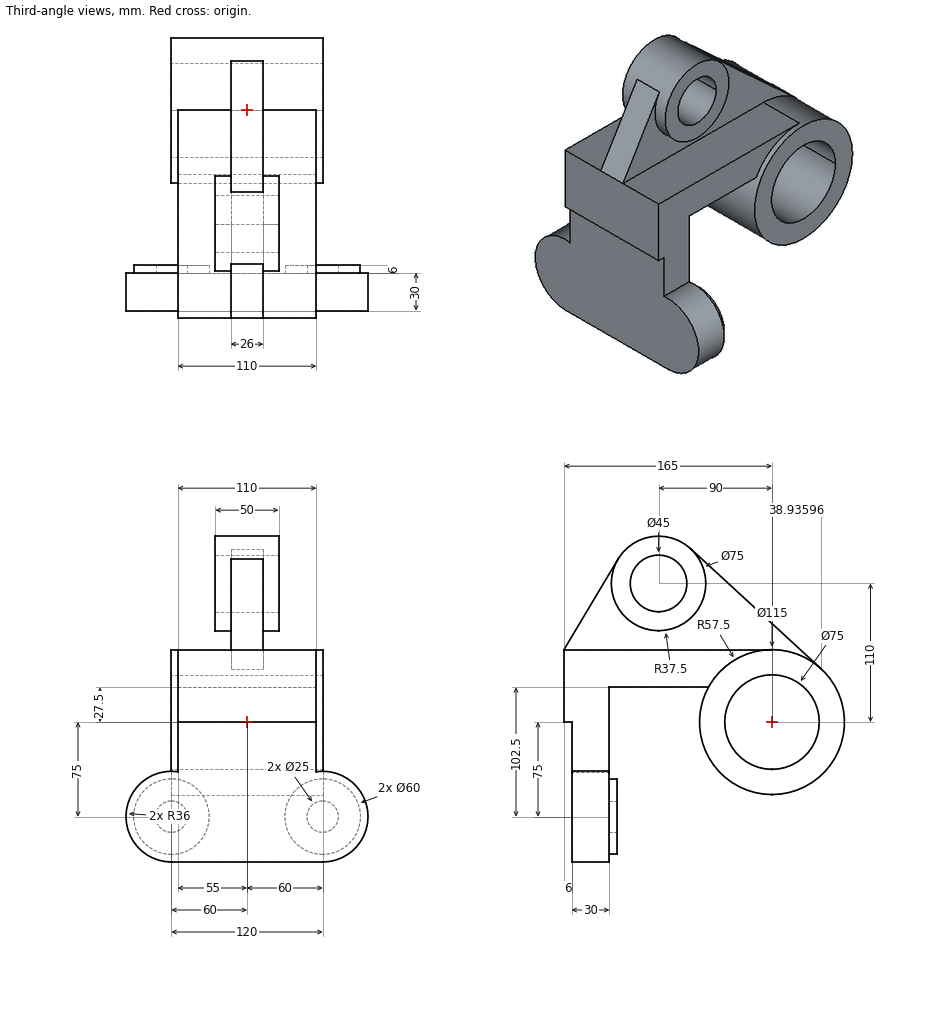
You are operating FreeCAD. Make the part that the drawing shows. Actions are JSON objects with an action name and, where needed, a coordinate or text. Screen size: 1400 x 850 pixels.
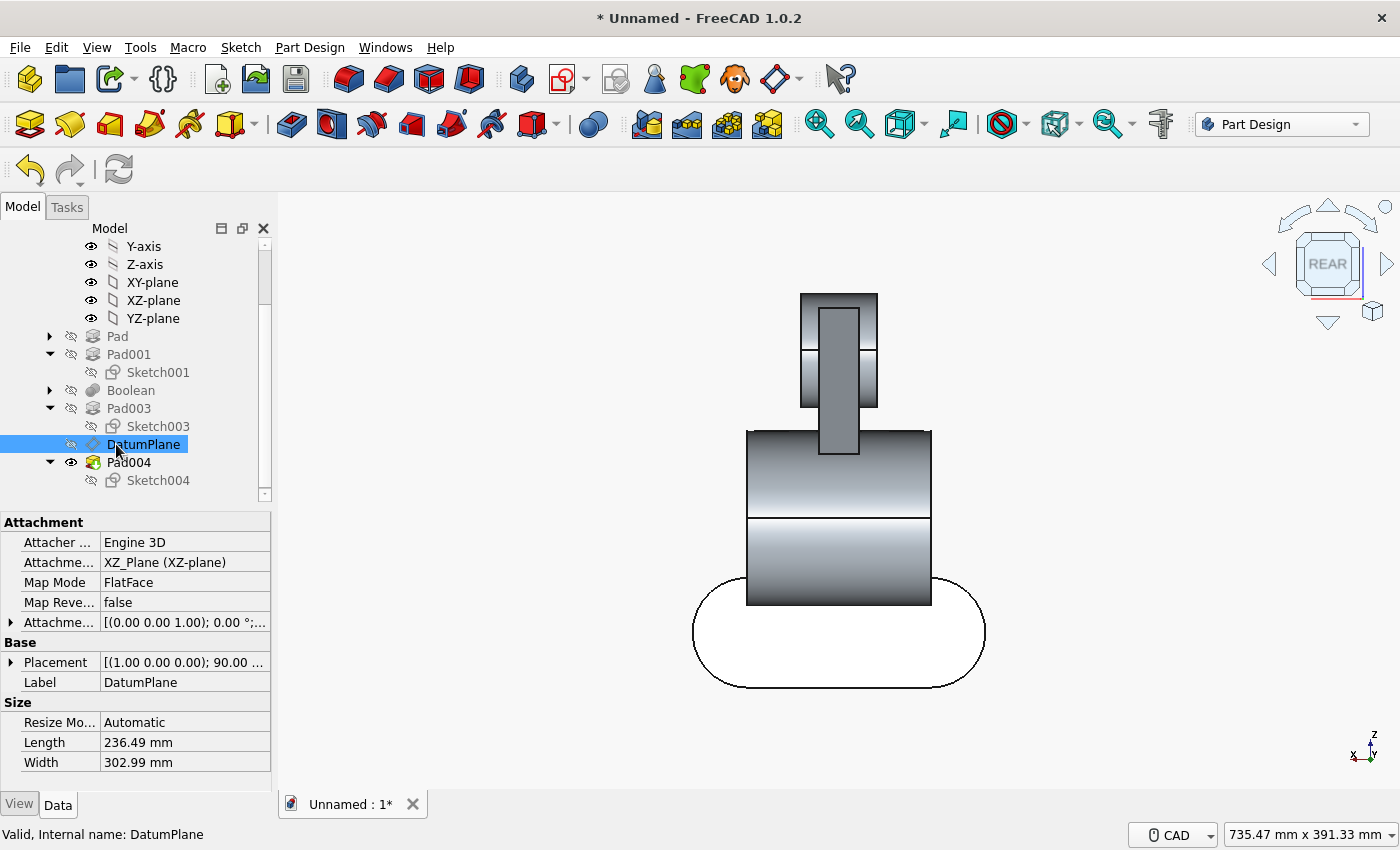
{"action": "left_click", "coordinate": [839, 611]}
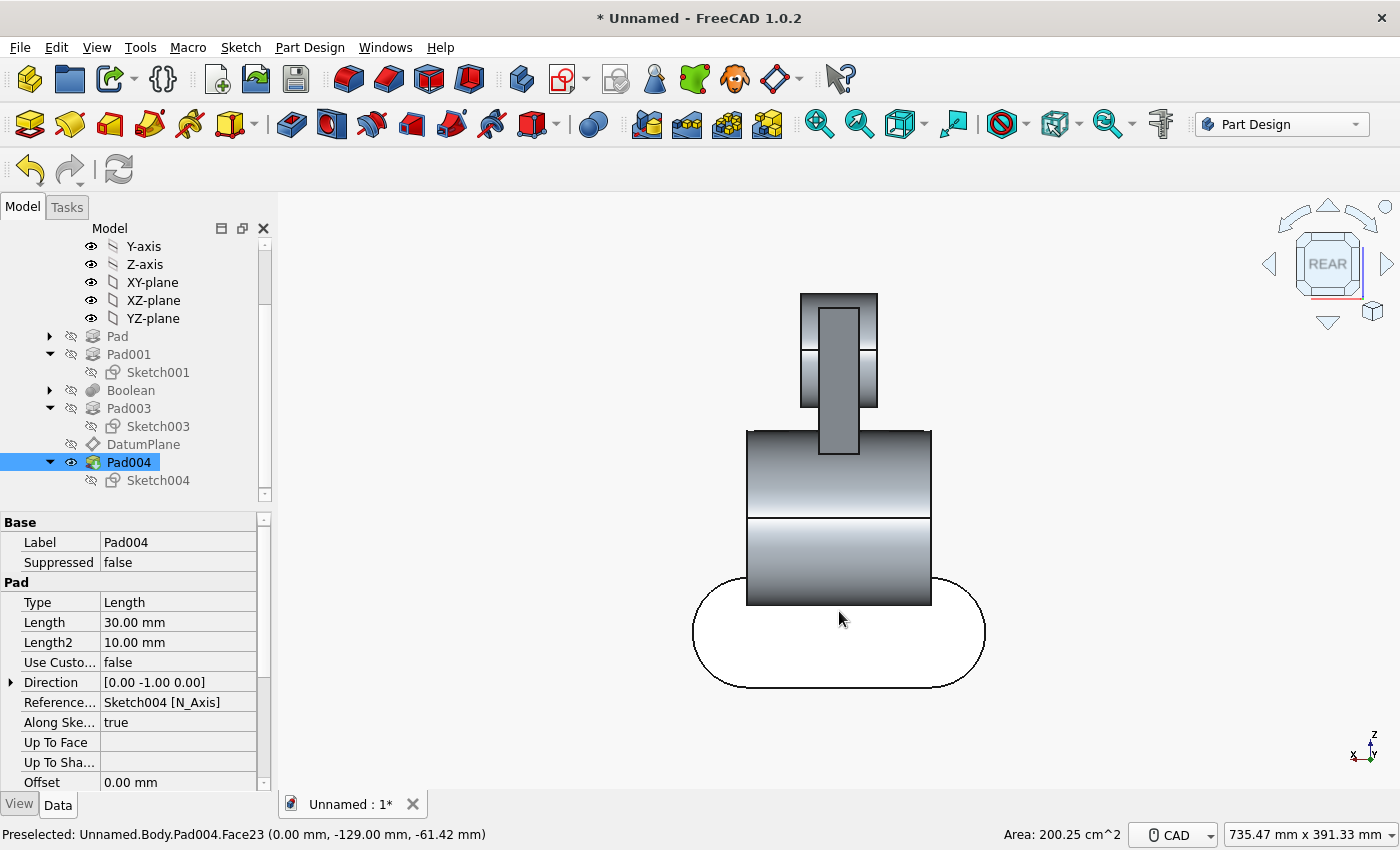
{"action": "left_click", "coordinate": [562, 80]}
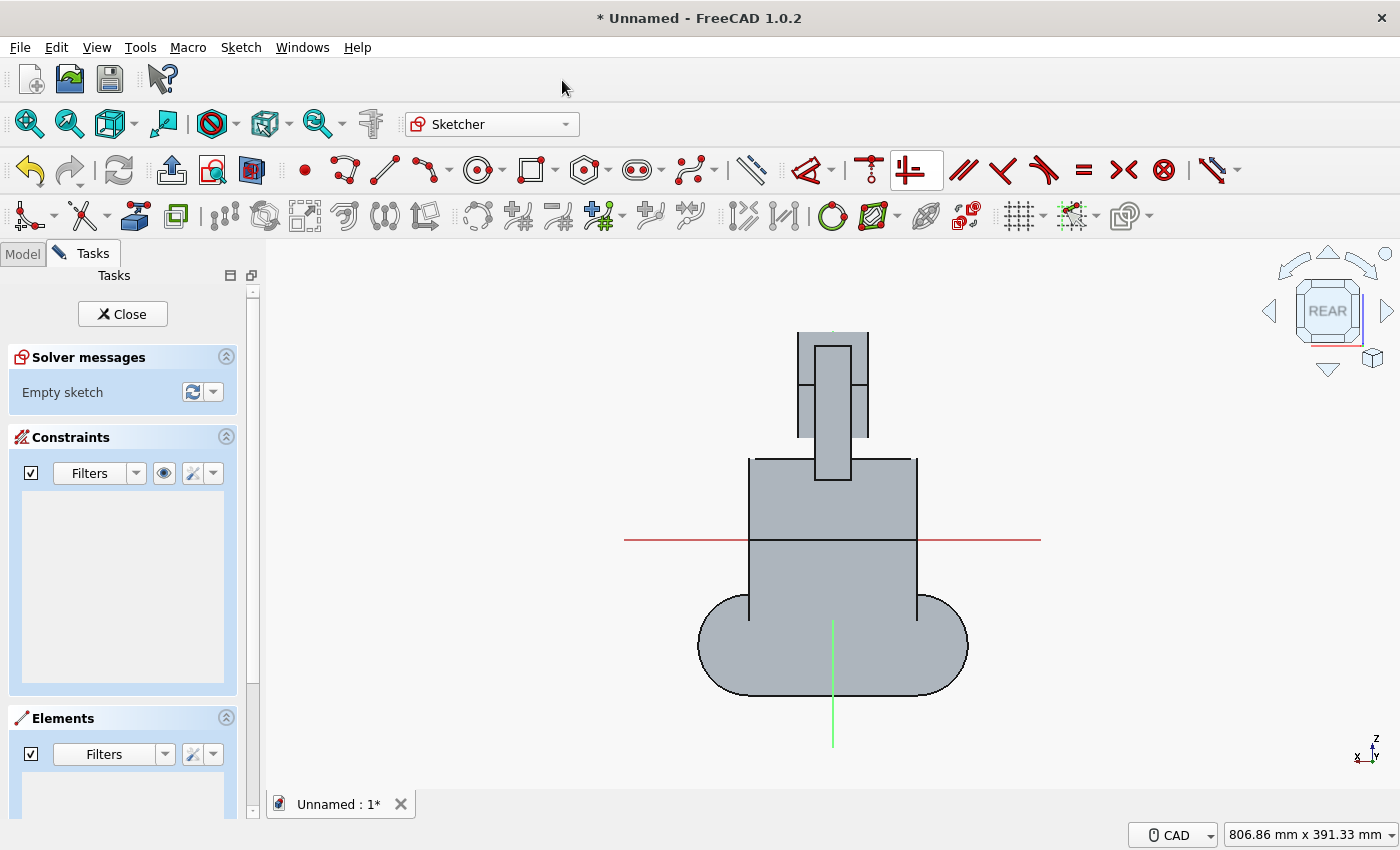
{"action": "scroll", "coordinate": [889, 695], "scroll_direction": "up", "scroll_amount": 4}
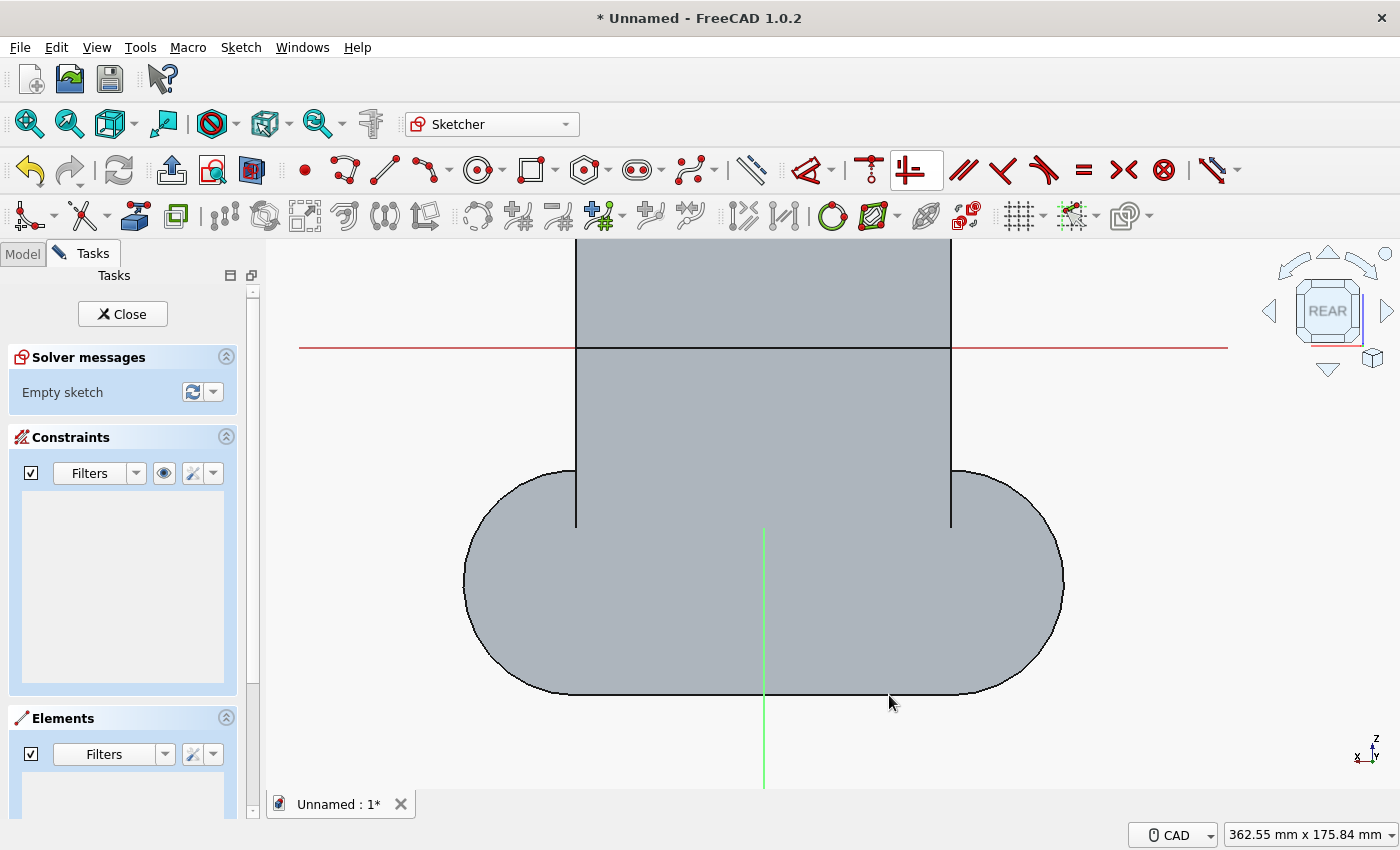
{"action": "left_click", "coordinate": [478, 170]}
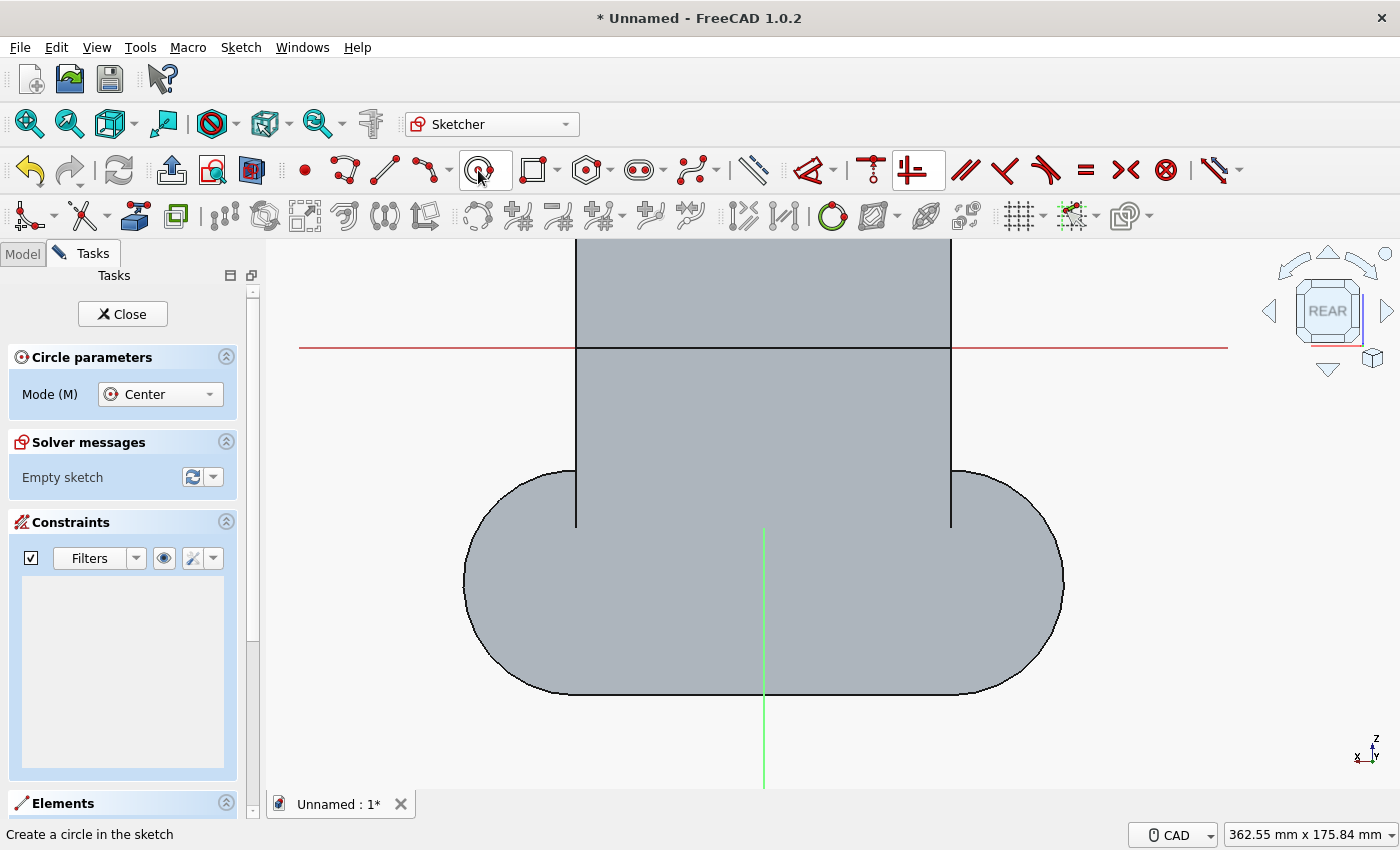
{"action": "left_click", "coordinate": [576, 583]}
{"action": "mouse_move", "coordinate": [642, 516]}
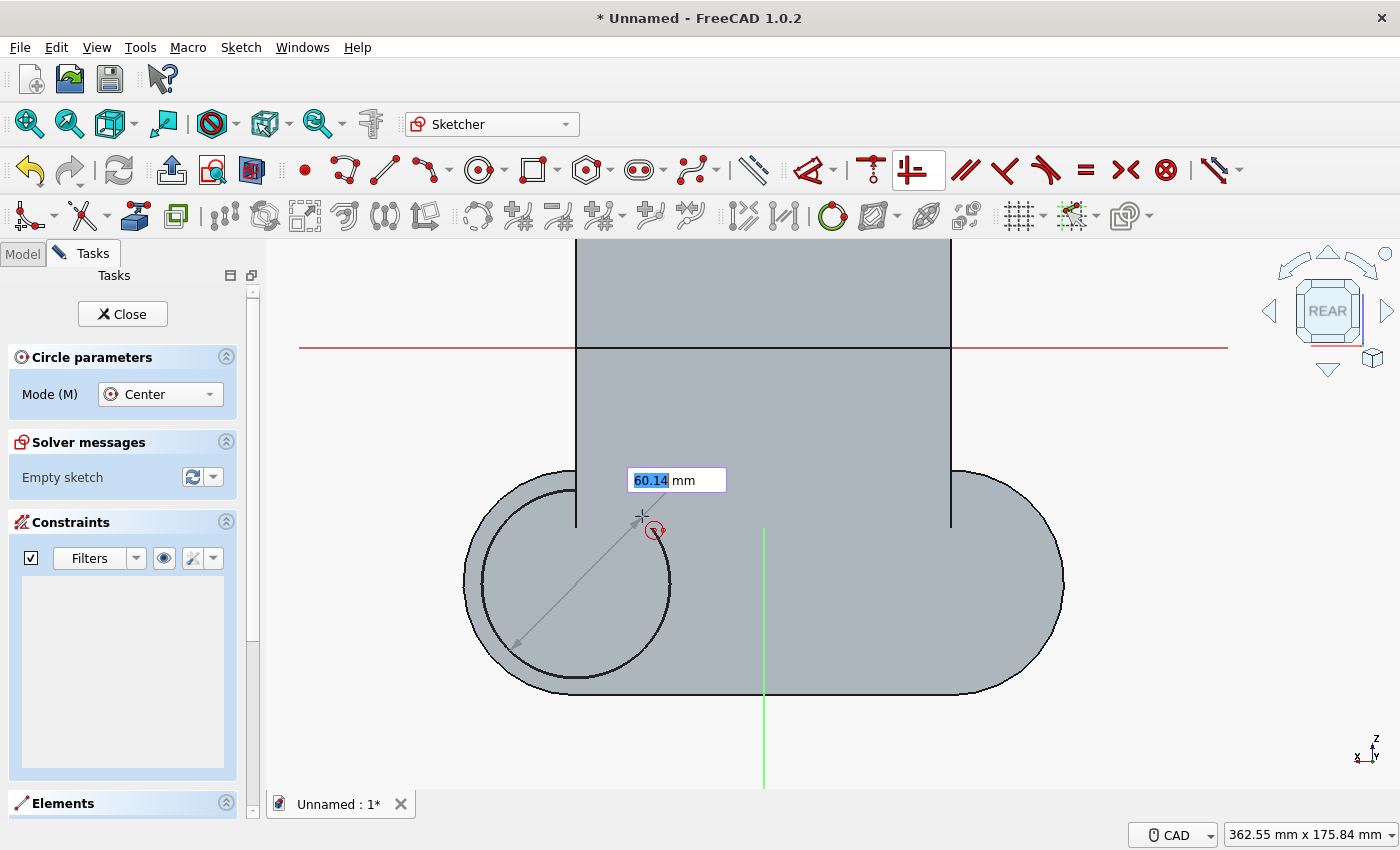
{"action": "type", "text": "60"}
{"action": "key", "text": "Return"}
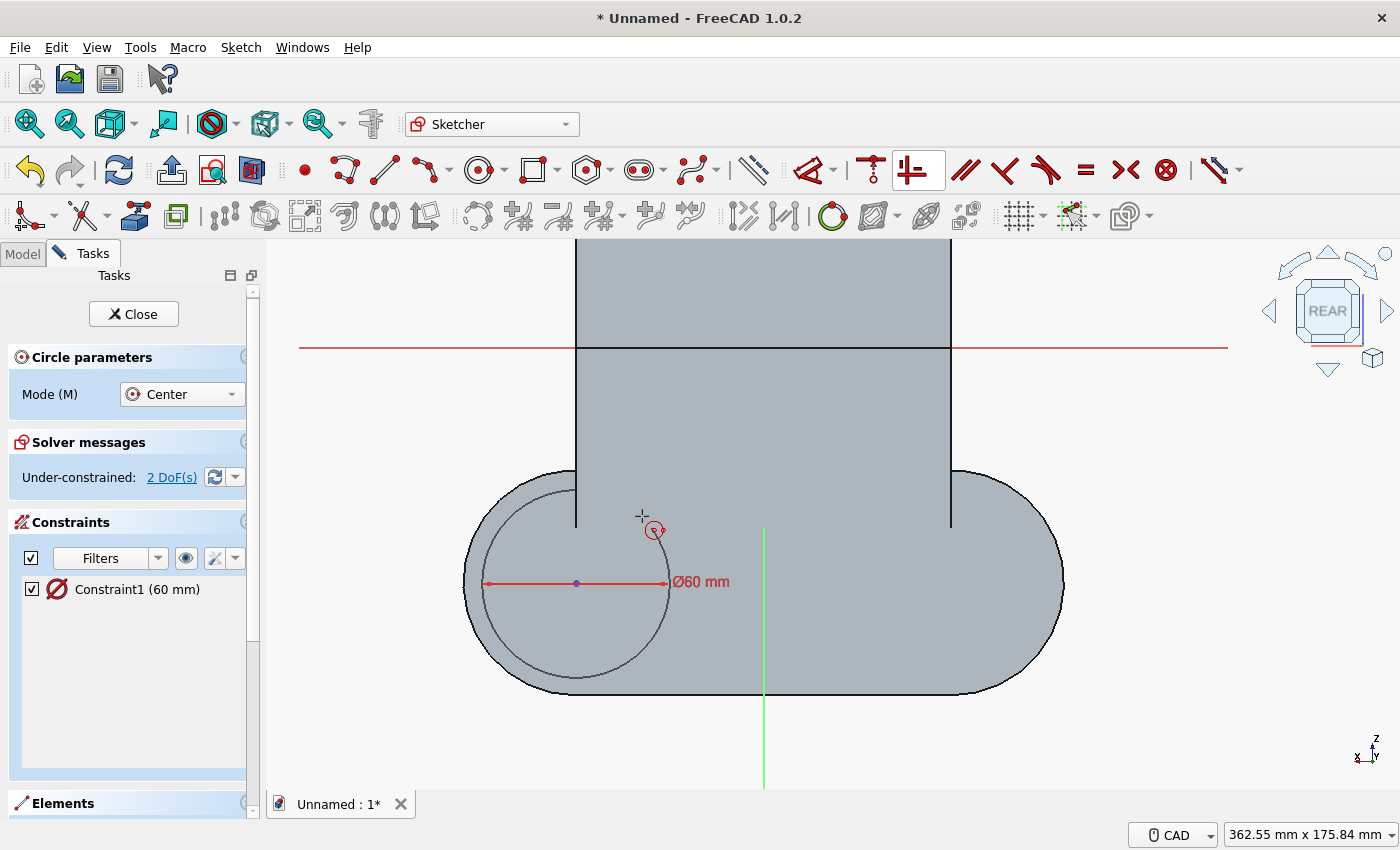
{"action": "left_click", "coordinate": [951, 583]}
{"action": "mouse_move", "coordinate": [1018, 516]}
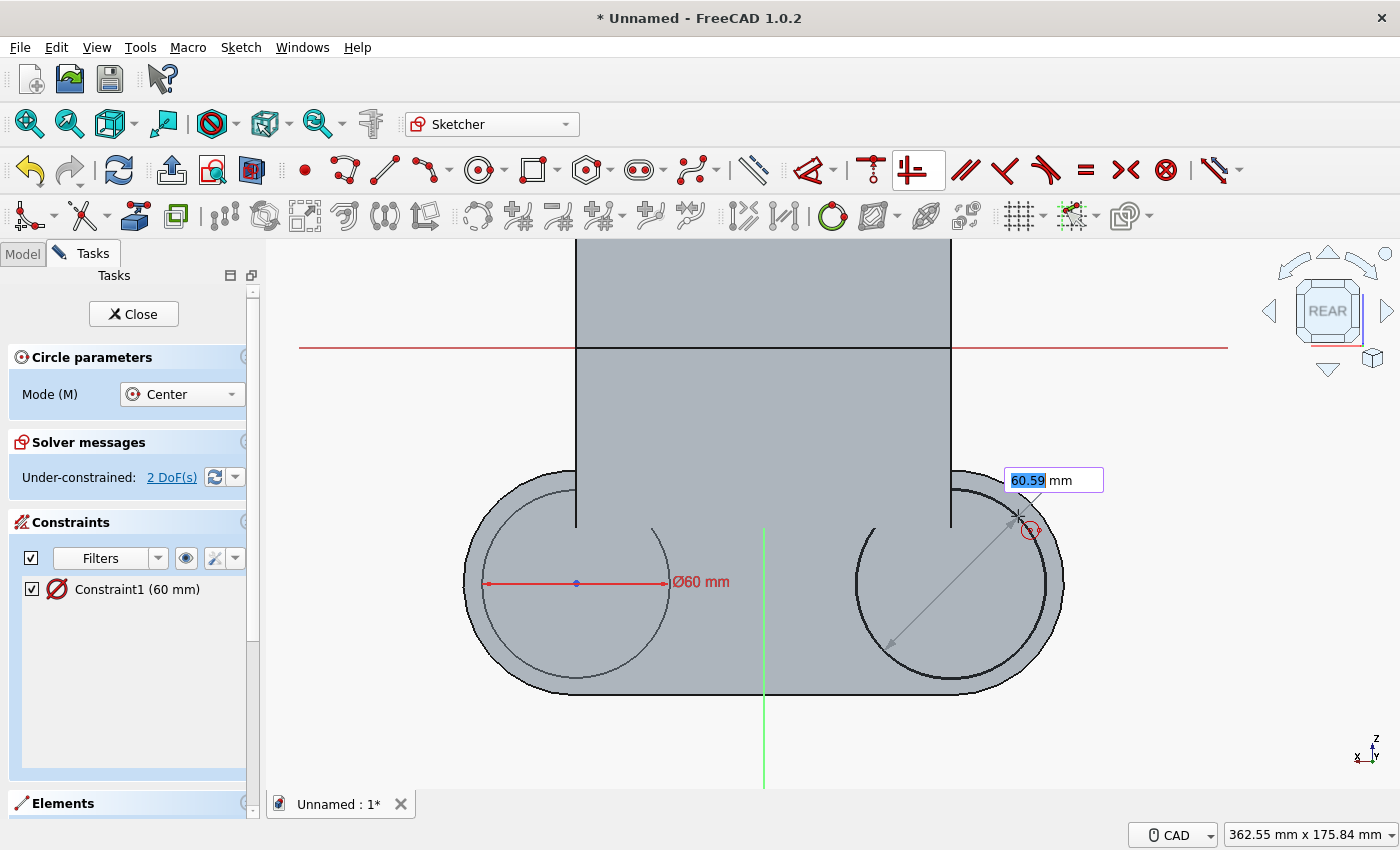
{"action": "type", "text": "60"}
{"action": "key", "text": "Return"}